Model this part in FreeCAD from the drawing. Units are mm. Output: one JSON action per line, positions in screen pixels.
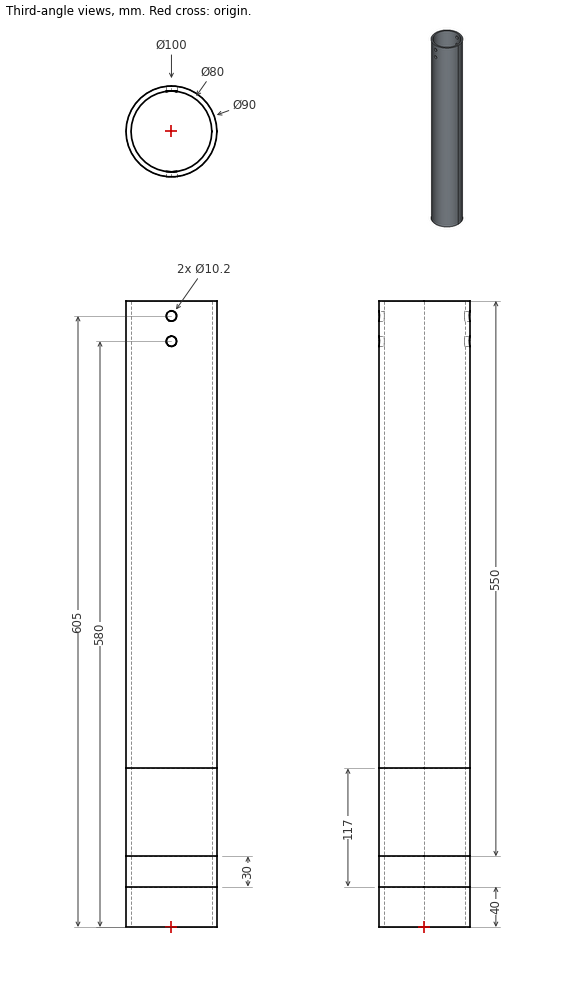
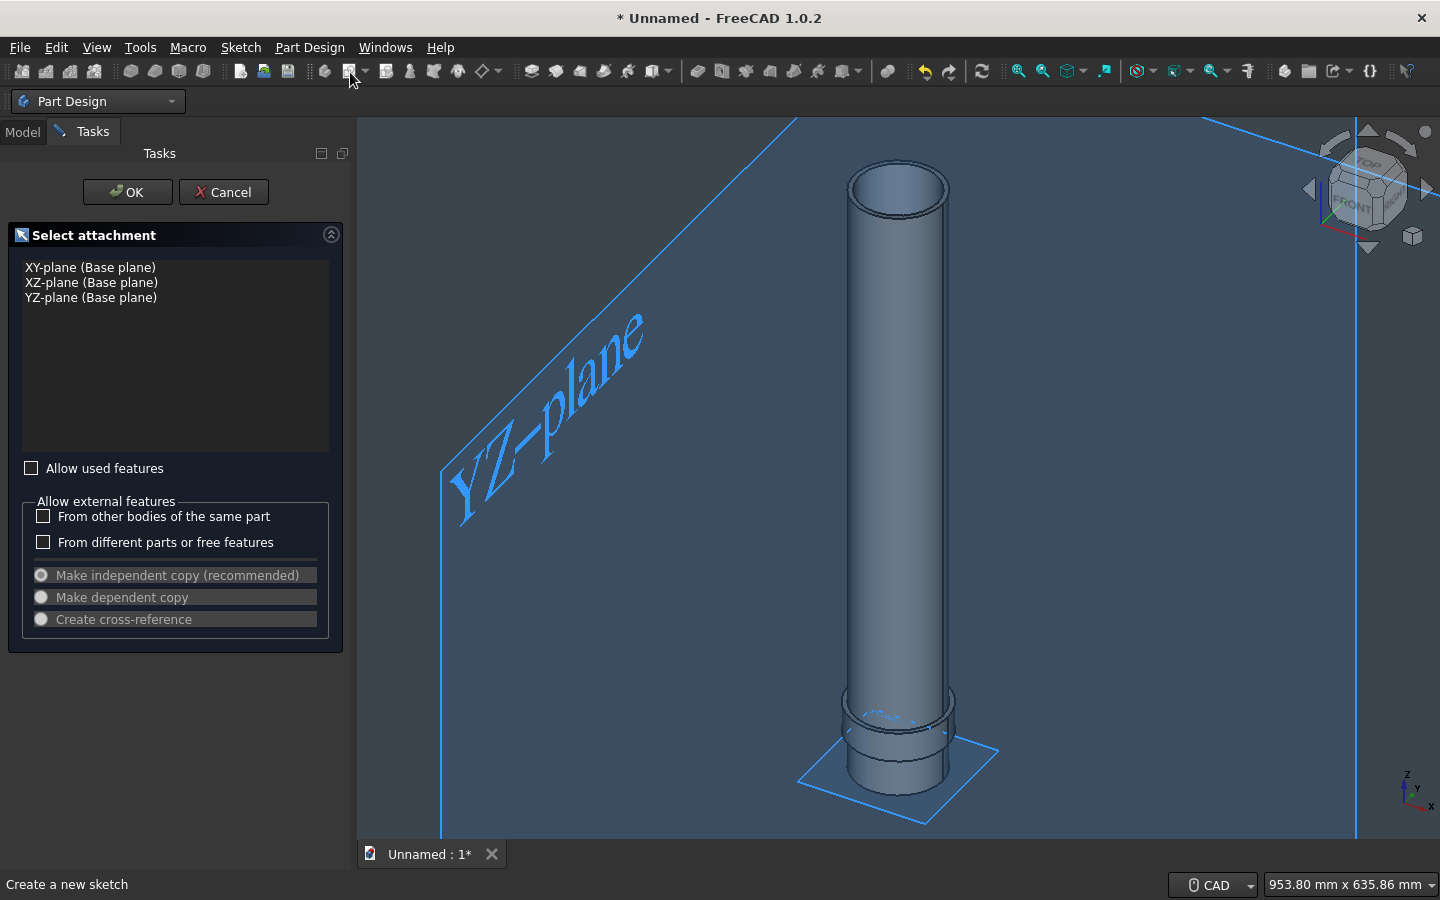
{"action": "left_click", "coordinate": [82, 282]}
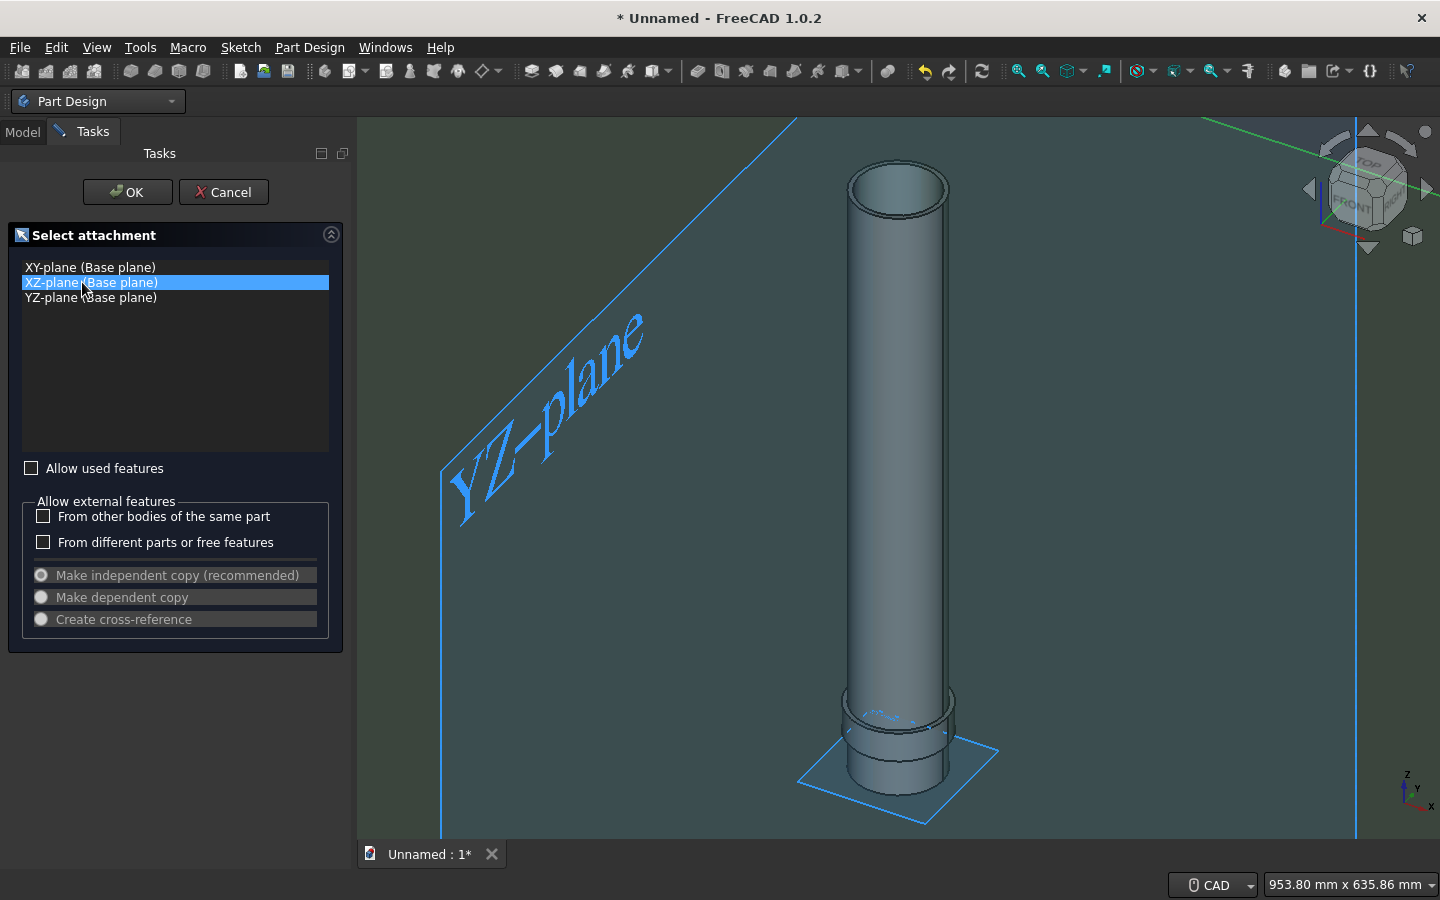
{"action": "left_click", "coordinate": [128, 192]}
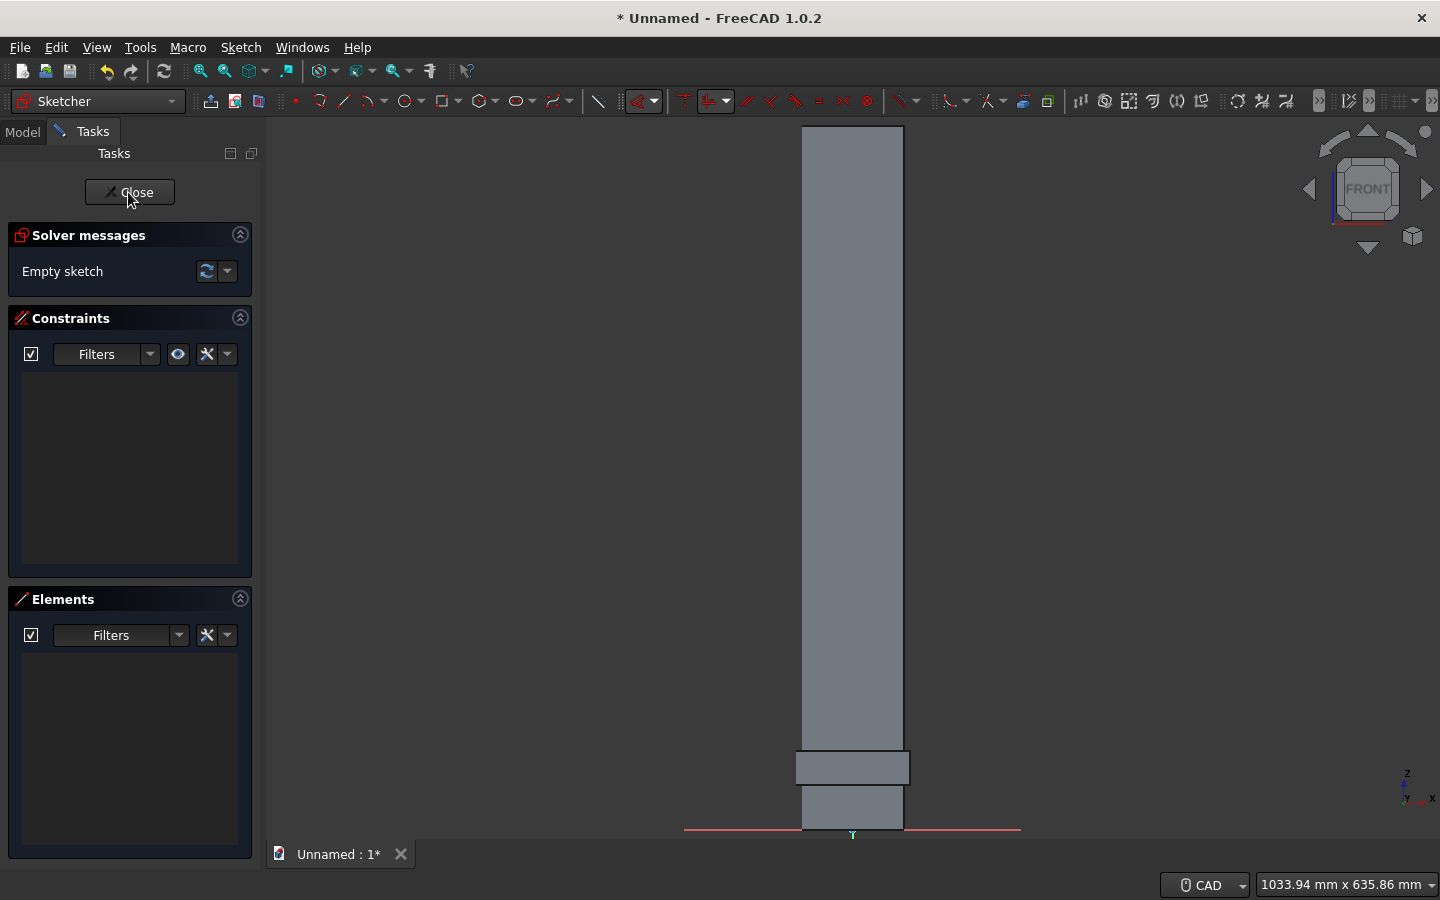
{"action": "left_click", "coordinate": [260, 102]}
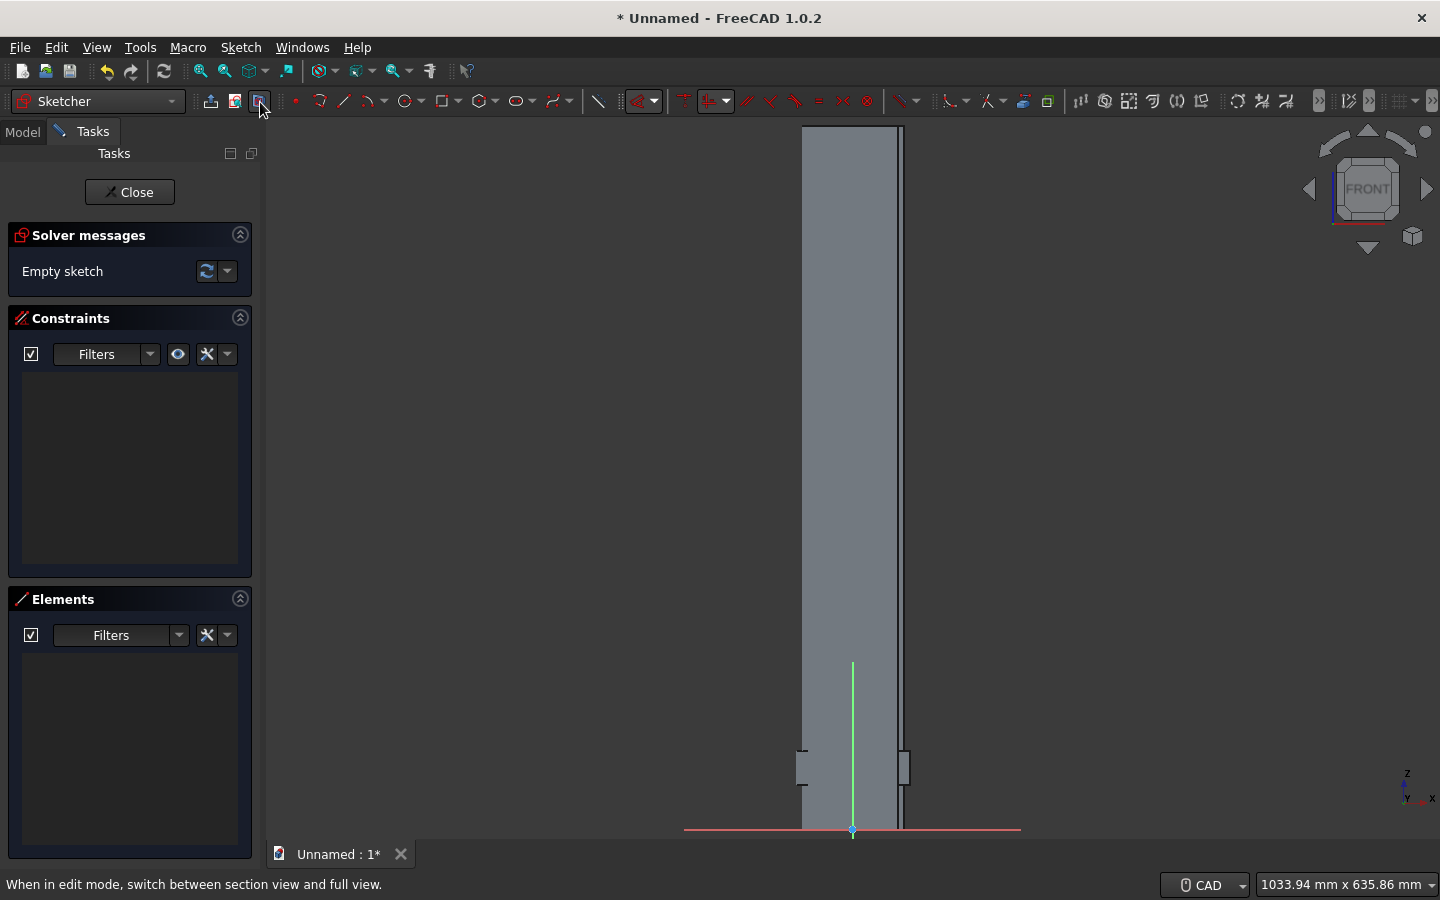
{"action": "scroll", "coordinate": [784, 478], "scroll_direction": "down", "scroll_amount": 5}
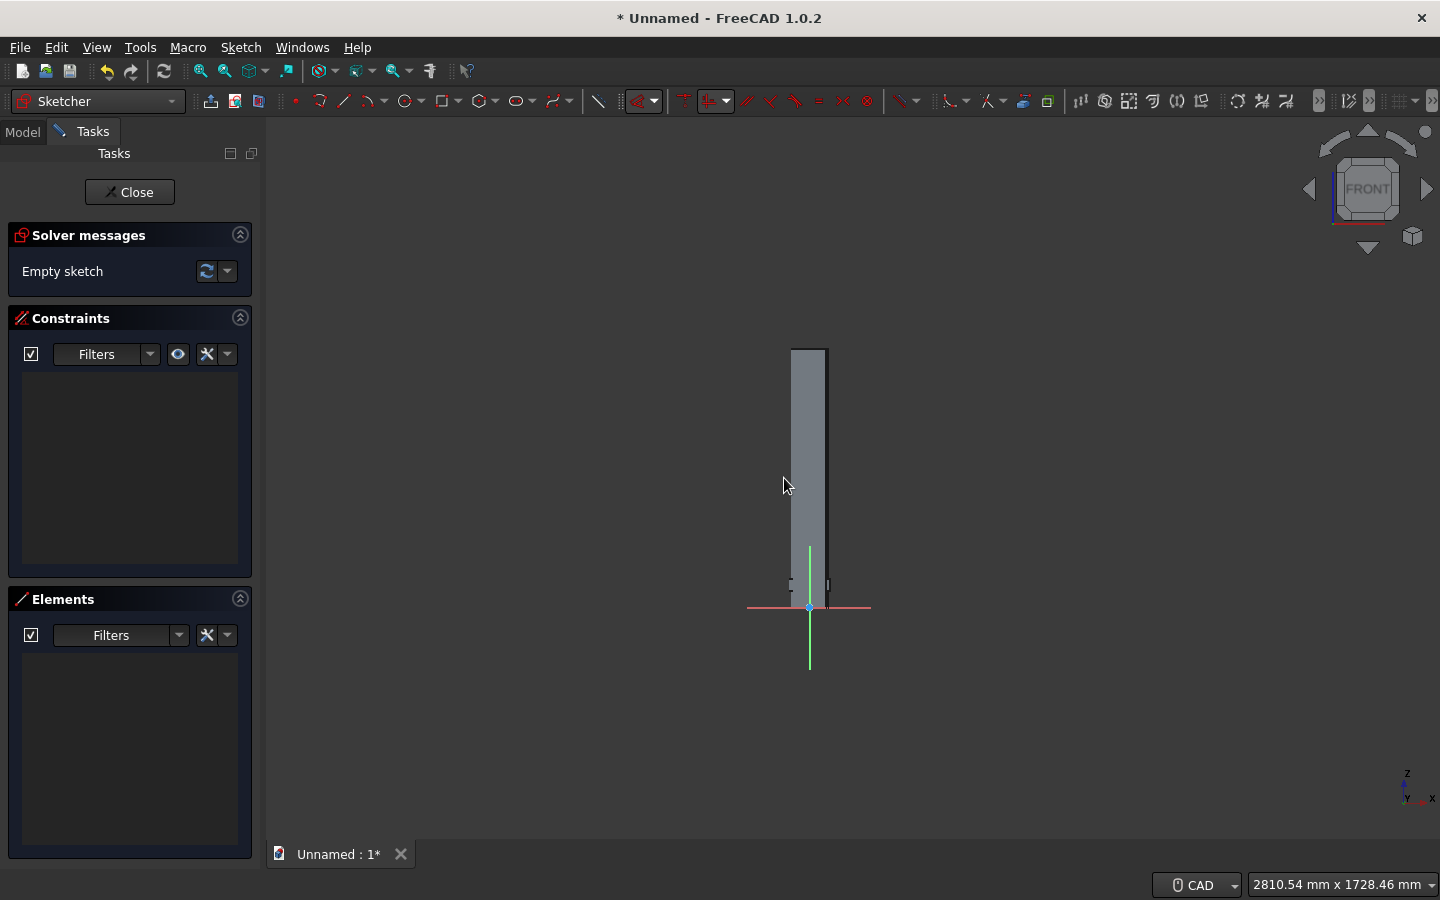
{"action": "scroll", "coordinate": [811, 354], "scroll_direction": "up", "scroll_amount": 15}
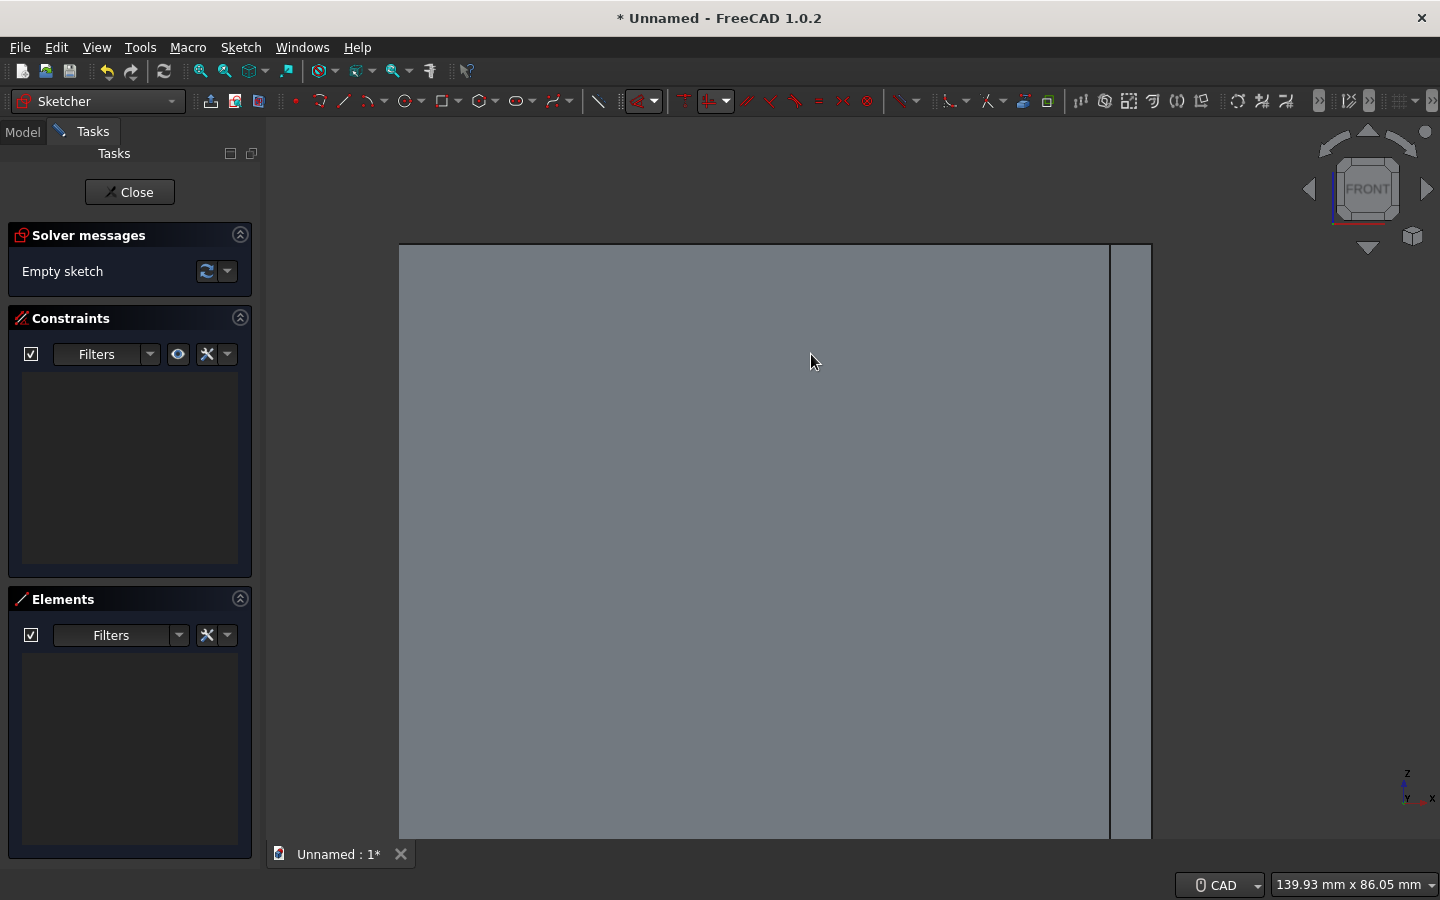
{"action": "scroll", "coordinate": [753, 467], "scroll_direction": "up", "scroll_amount": 2}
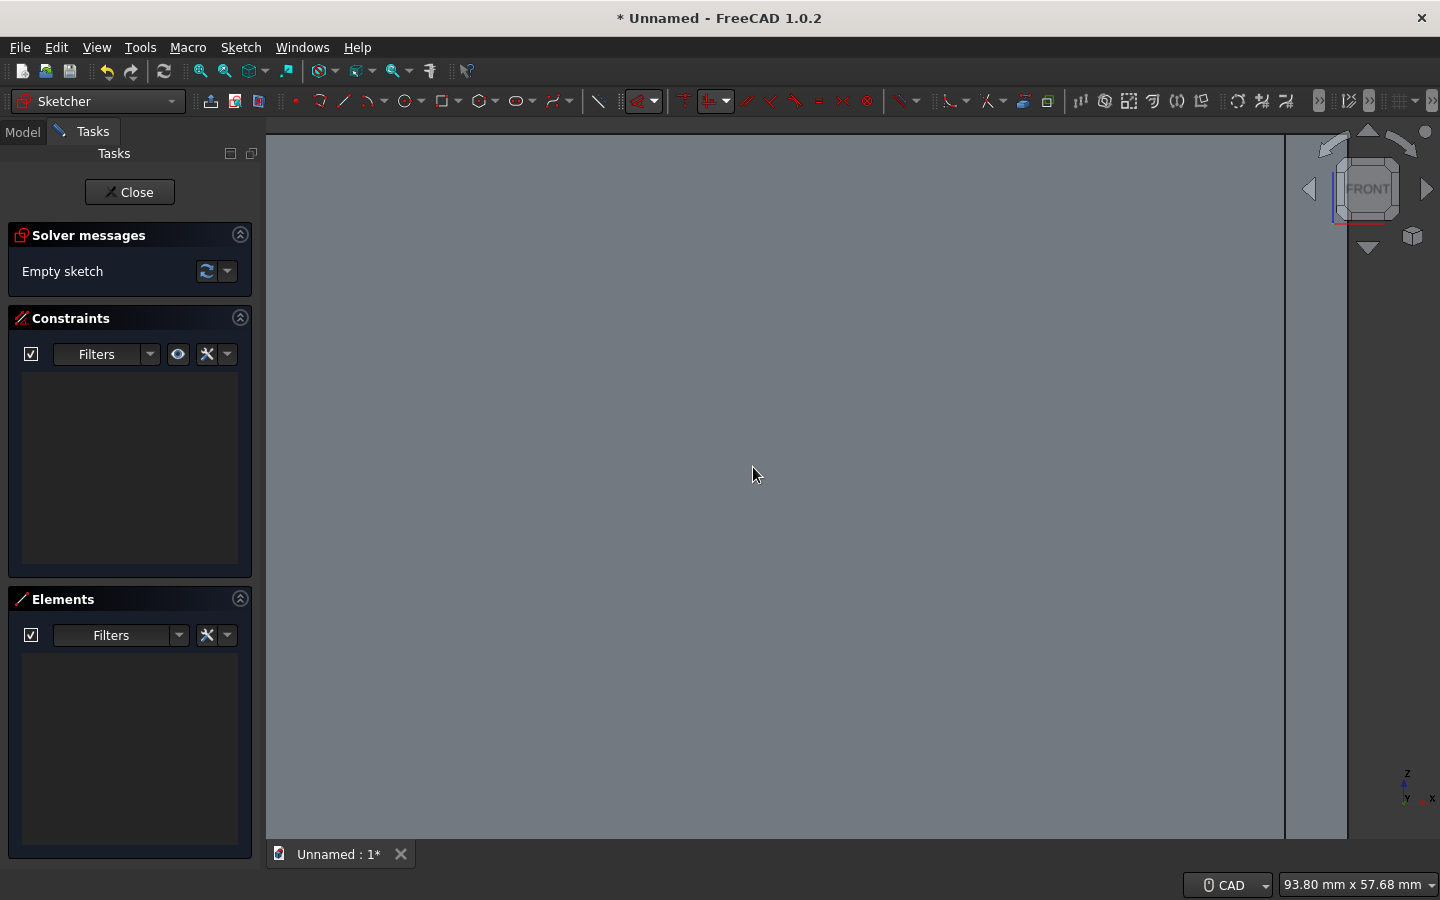
{"action": "key", "text": "g c"}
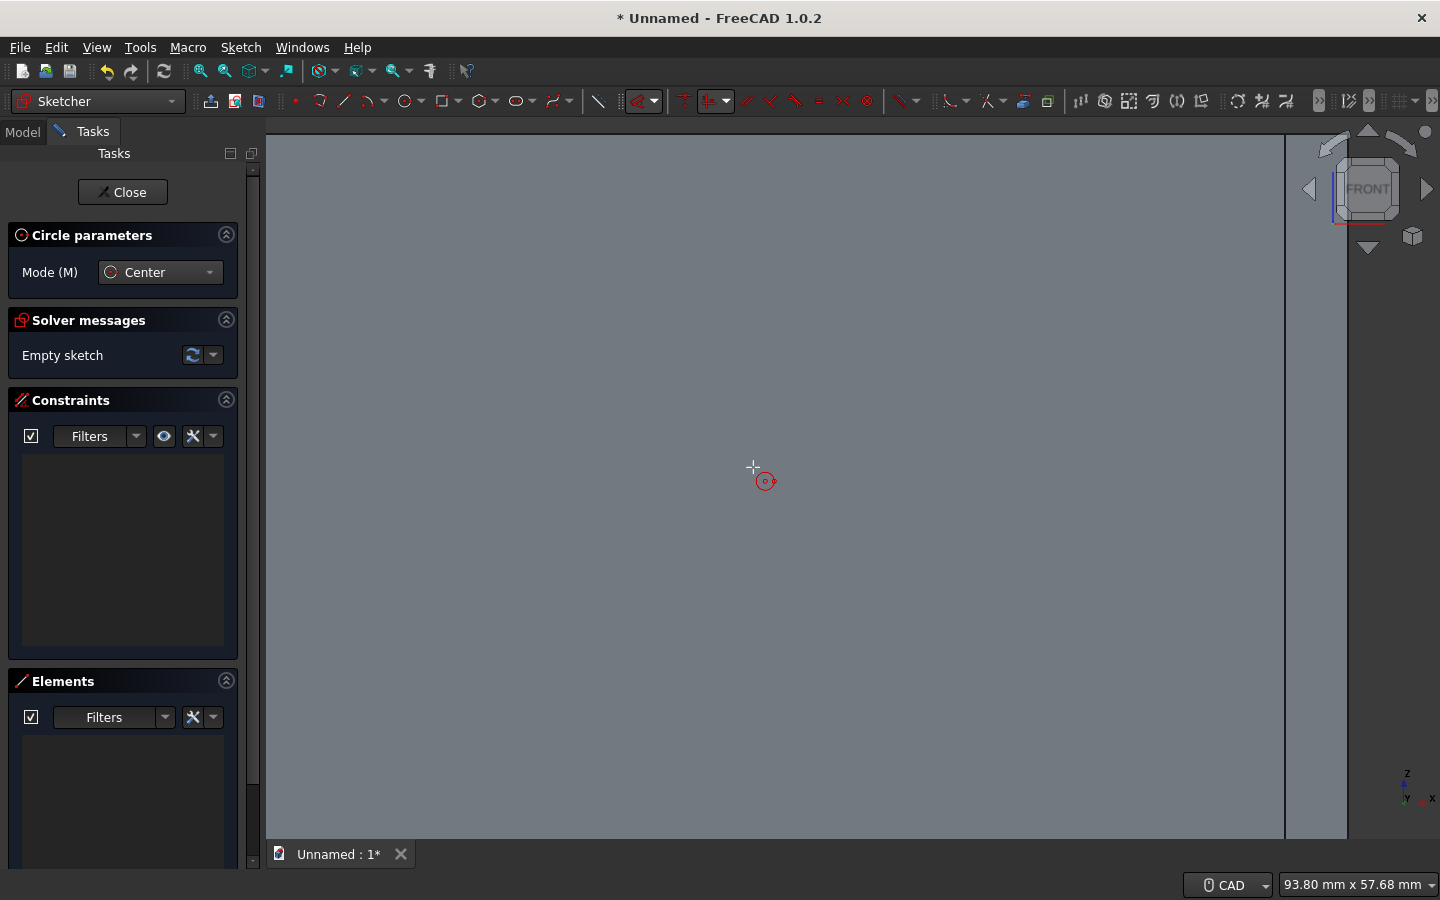
{"action": "left_click", "coordinate": [784, 322]}
{"action": "mouse_move", "coordinate": [830, 276]}